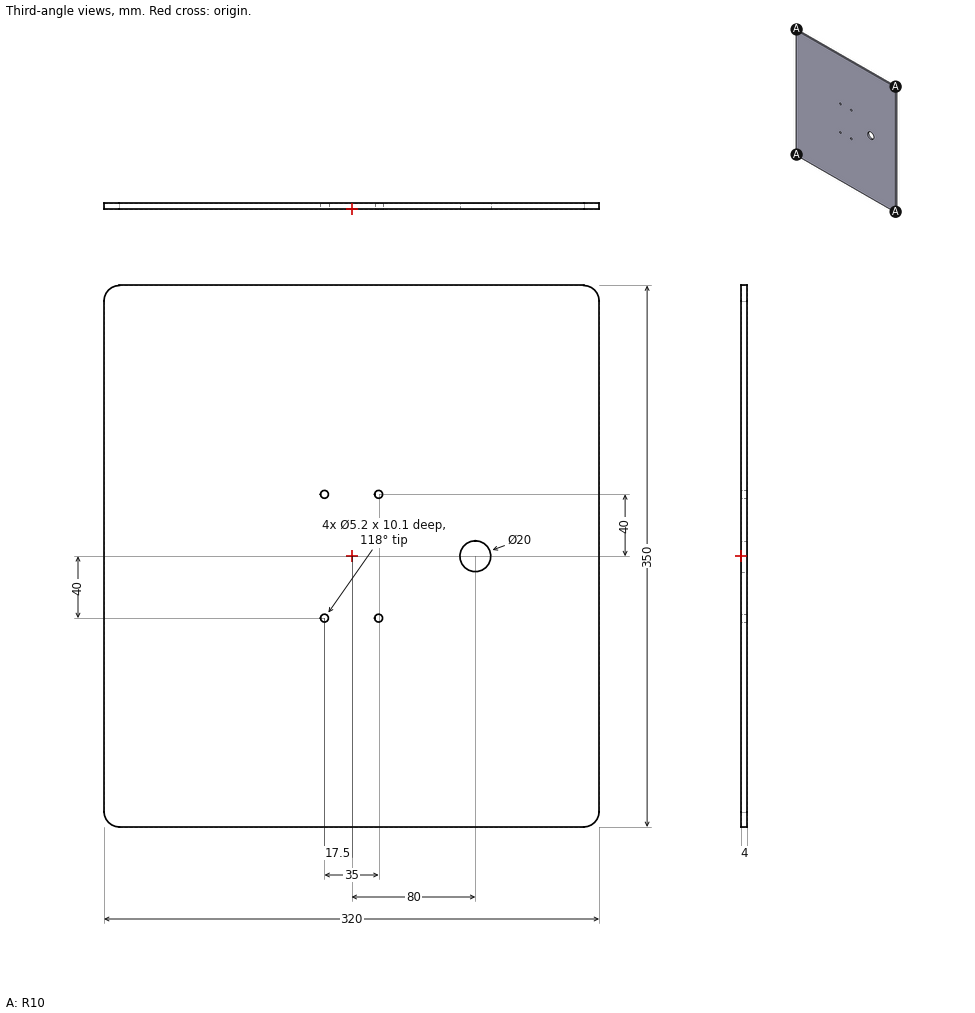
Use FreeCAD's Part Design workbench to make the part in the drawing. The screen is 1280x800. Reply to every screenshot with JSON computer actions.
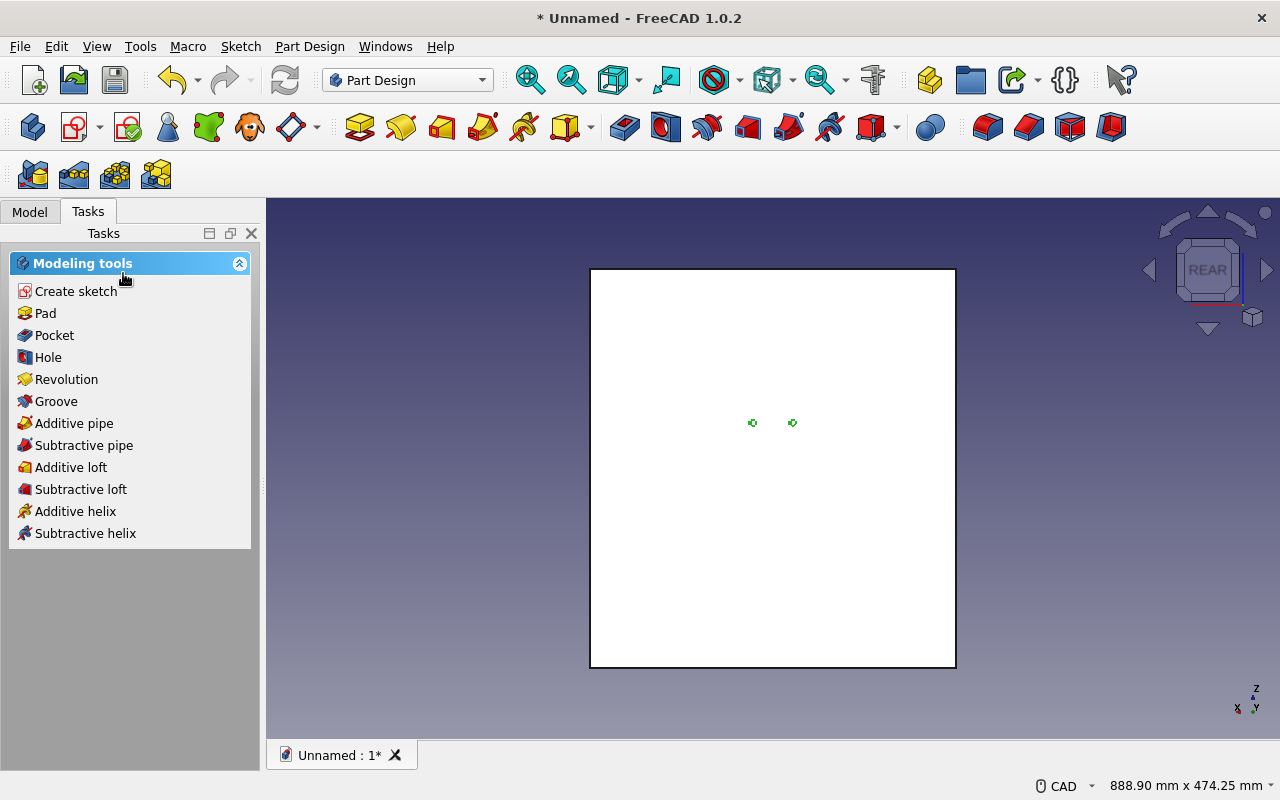
{"action": "left_click", "coordinate": [666, 128]}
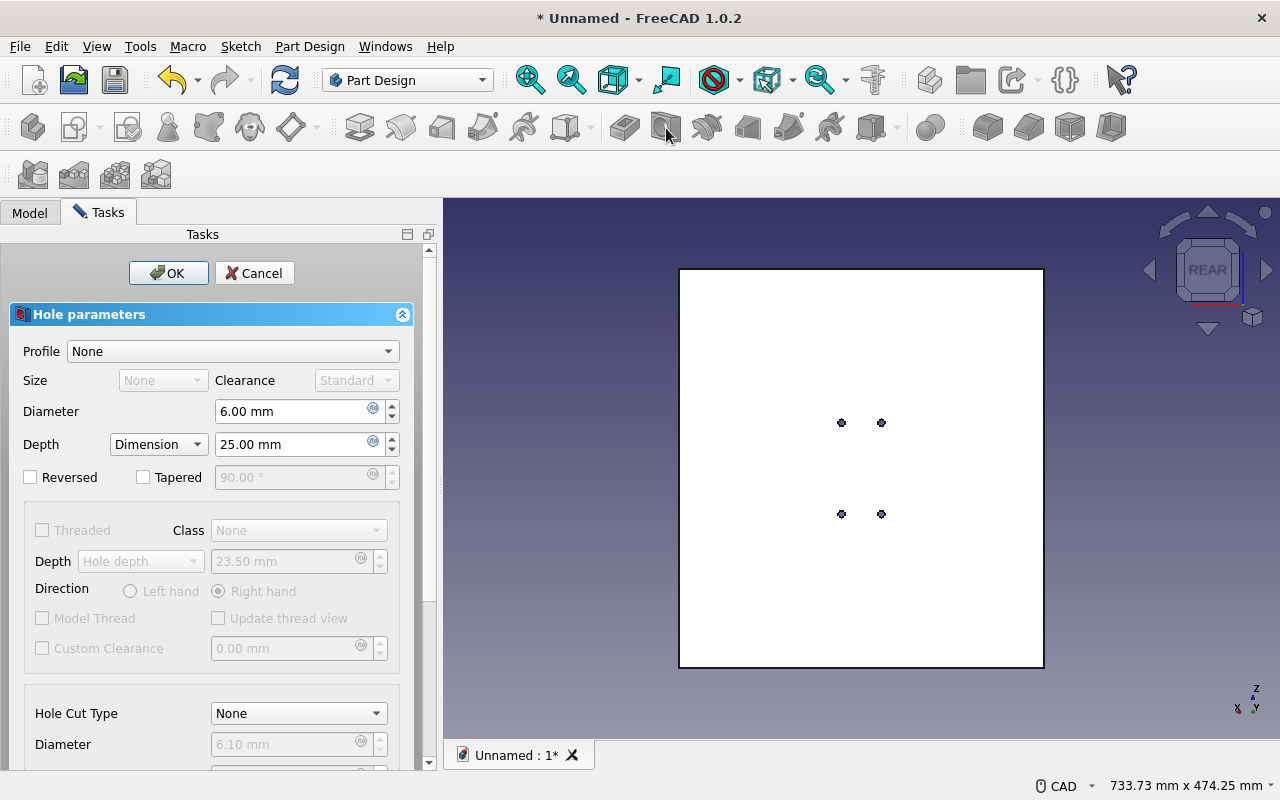
{"action": "triple_click", "coordinate": [300, 412]}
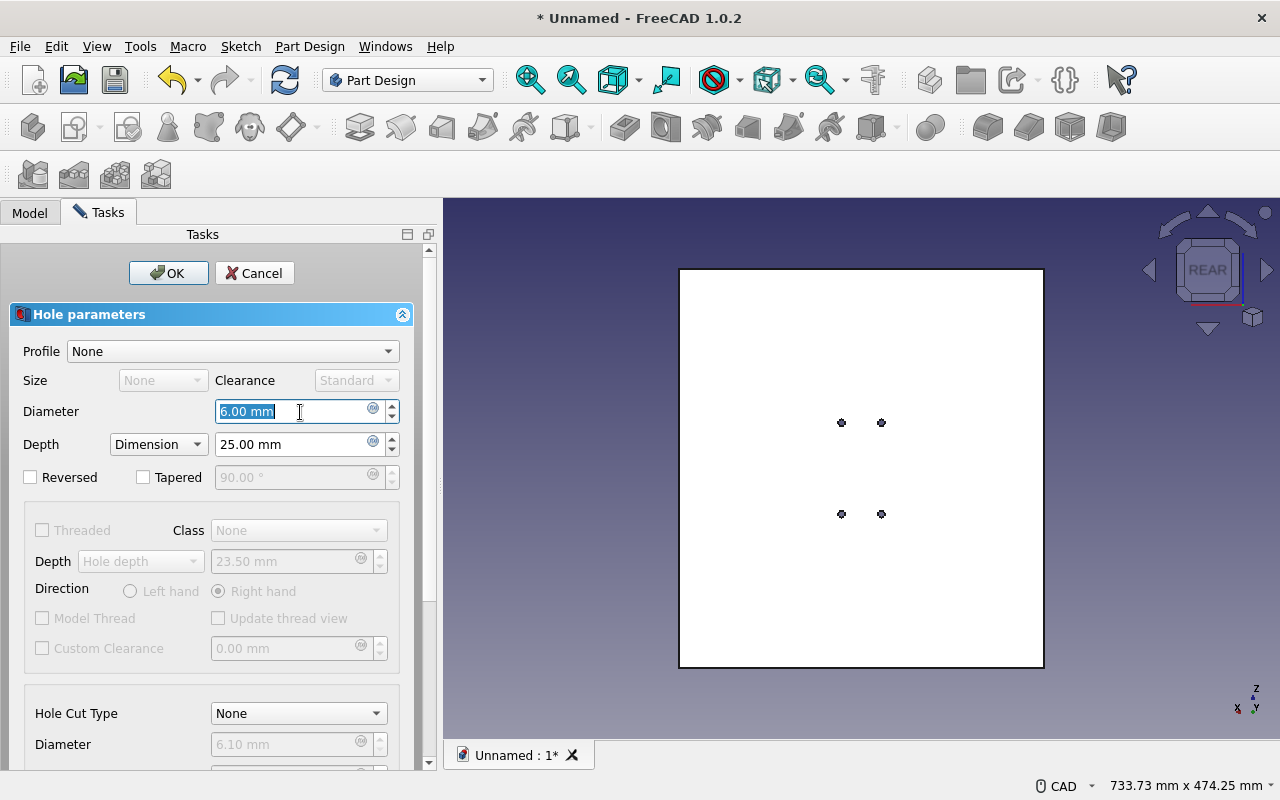
{"action": "type", "text": "5.2"}
{"action": "key", "text": "Tab"}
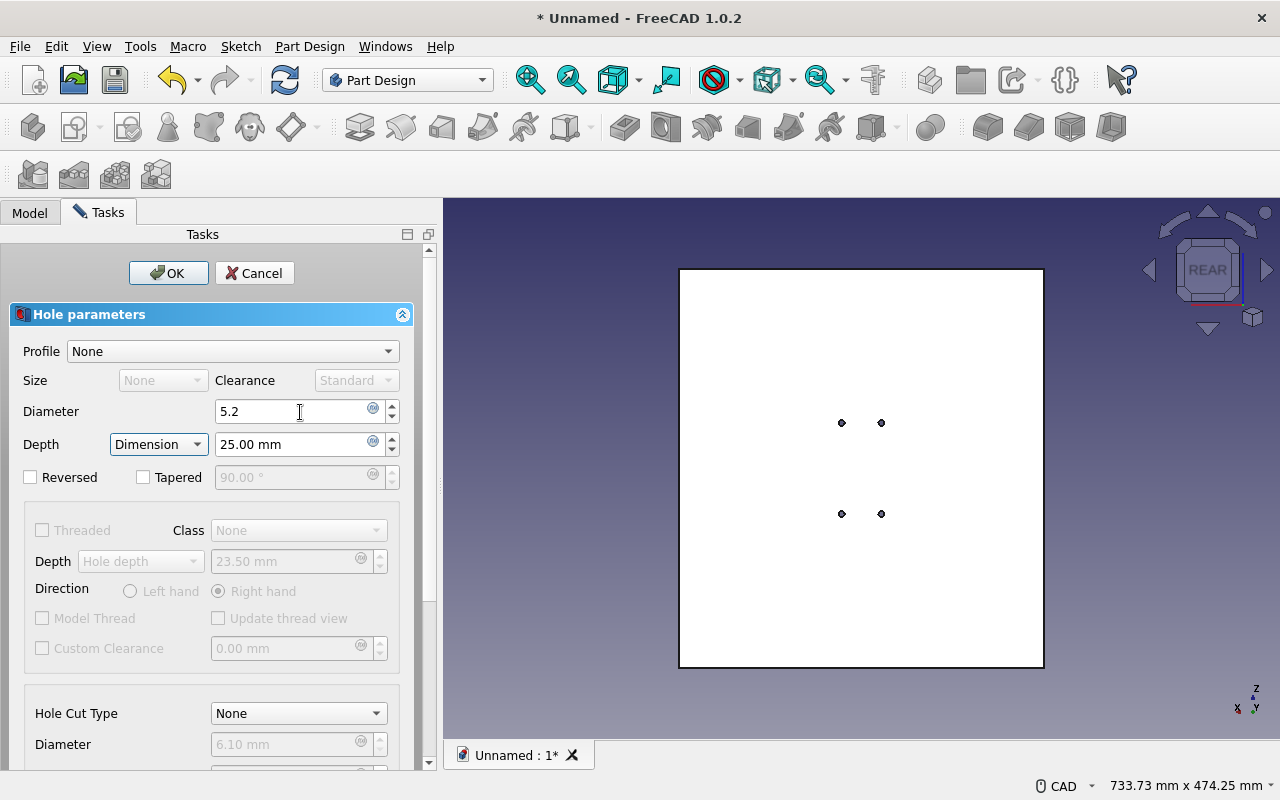
{"action": "triple_click", "coordinate": [300, 444]}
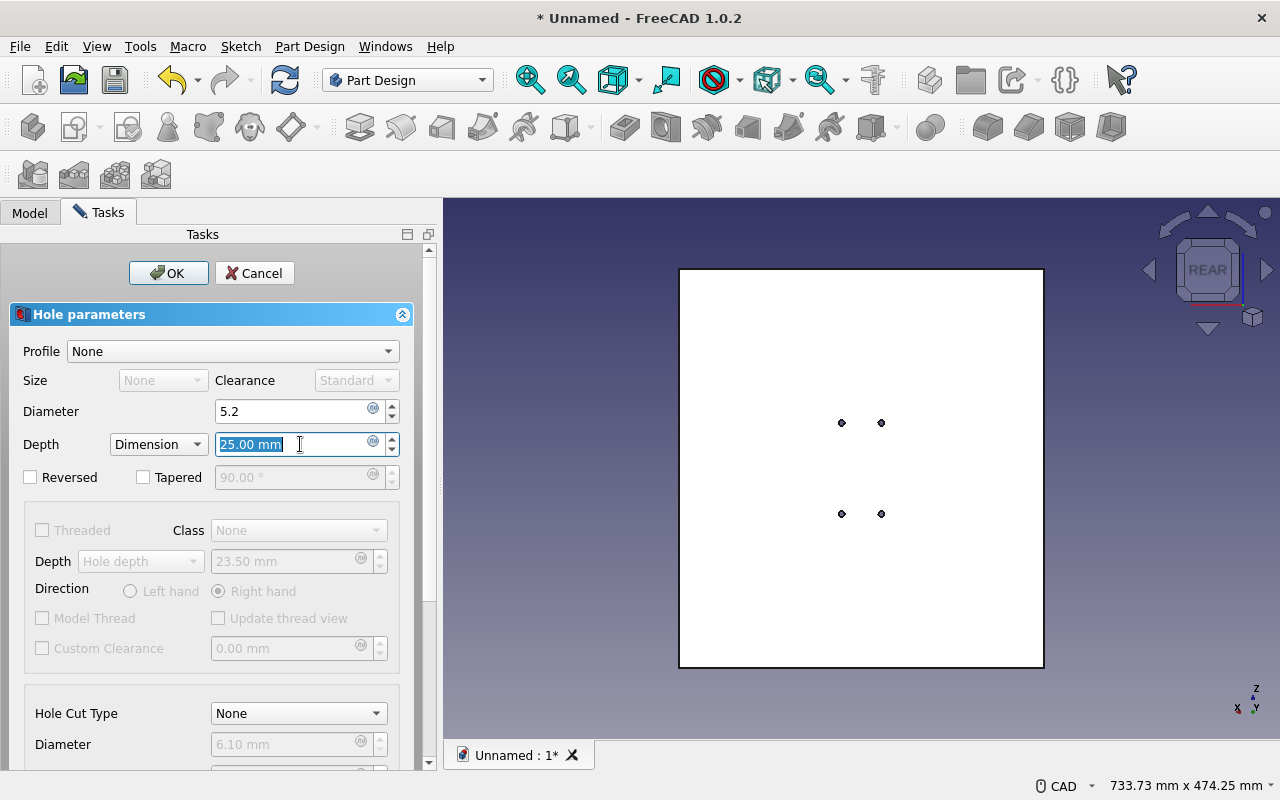
{"action": "type", "text": "10.1"}
{"action": "key", "text": "Tab"}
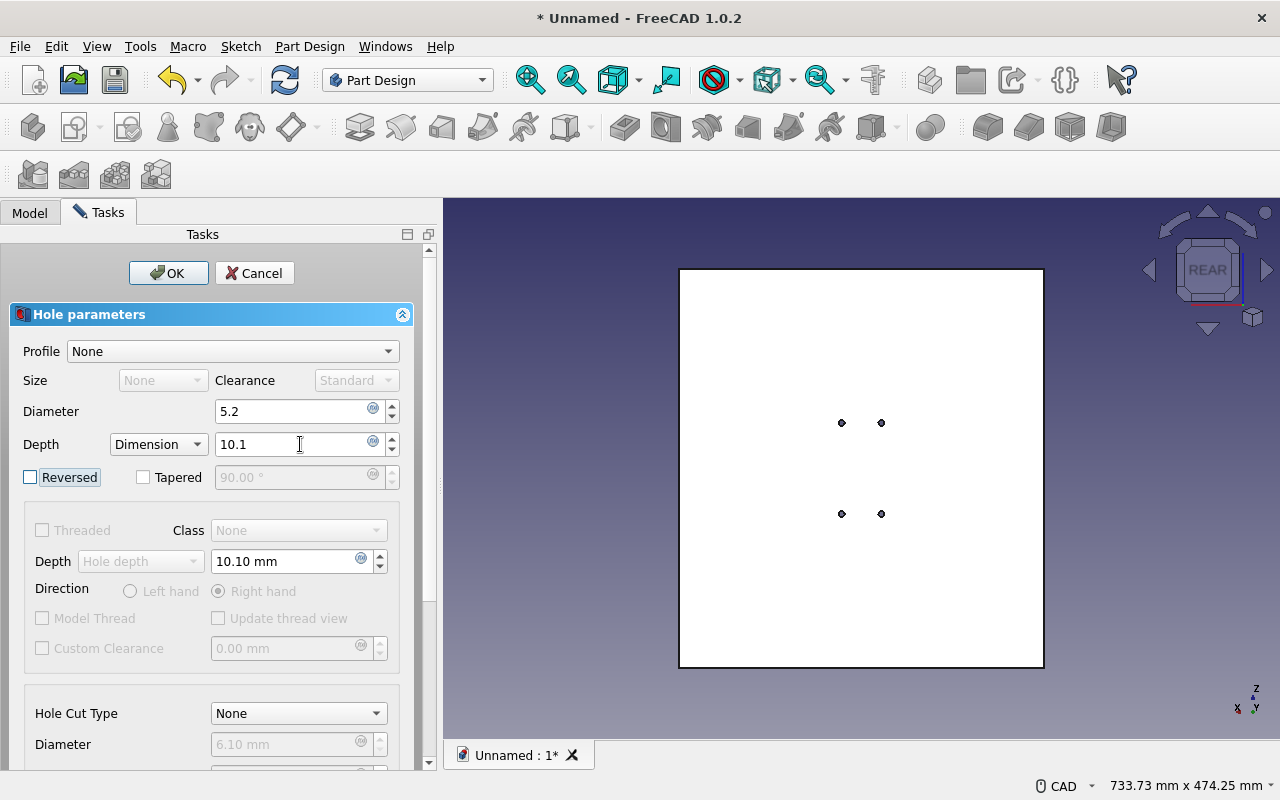
{"action": "left_click", "coordinate": [169, 273]}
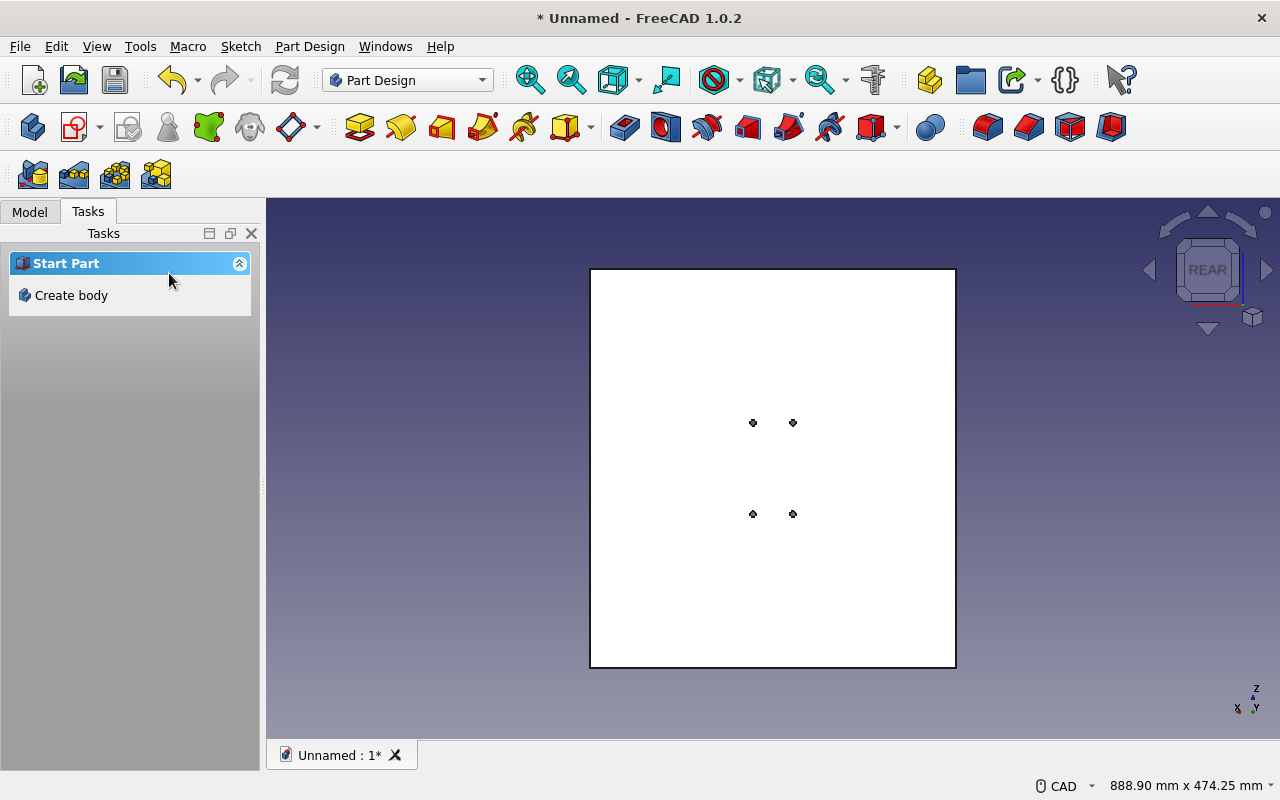
{"action": "scroll", "coordinate": [956, 667], "scroll_direction": "up", "scroll_amount": 11}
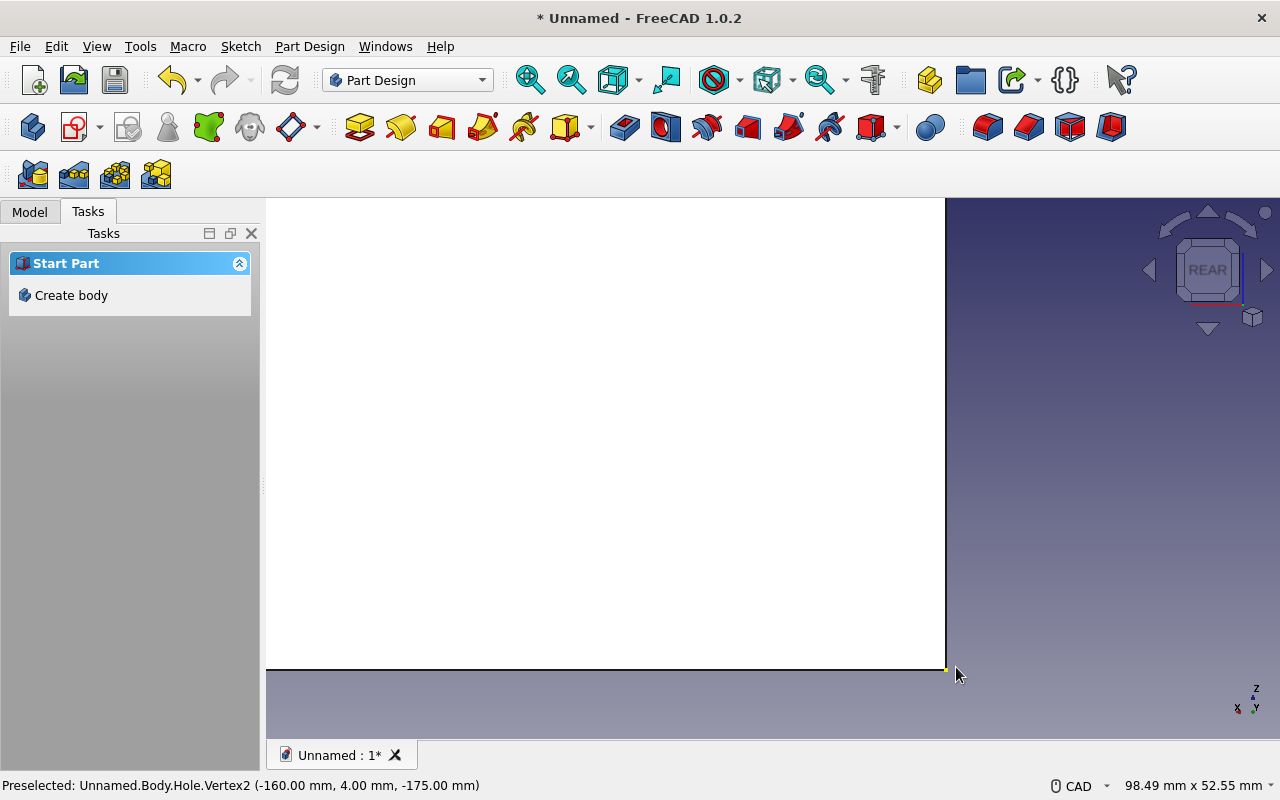
{"action": "left_click", "coordinate": [531, 80]}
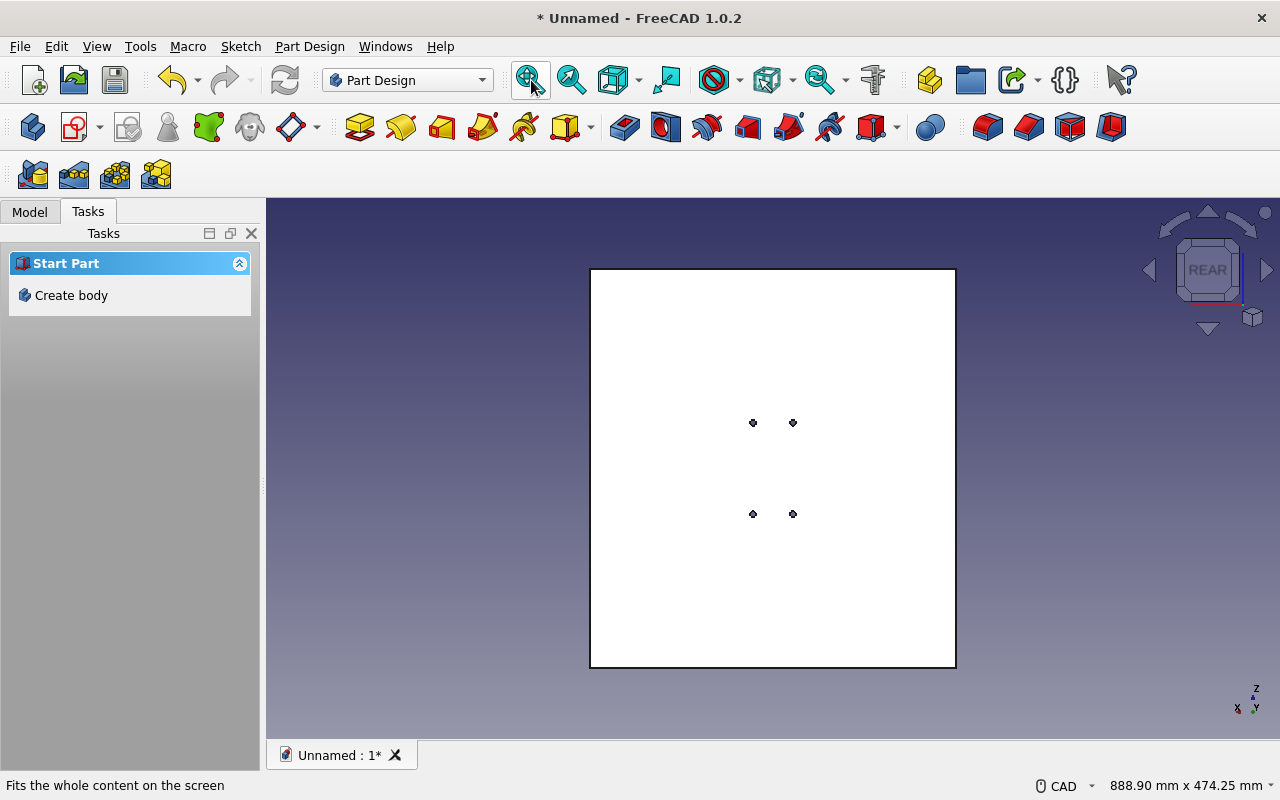
{"action": "key", "text": "0"}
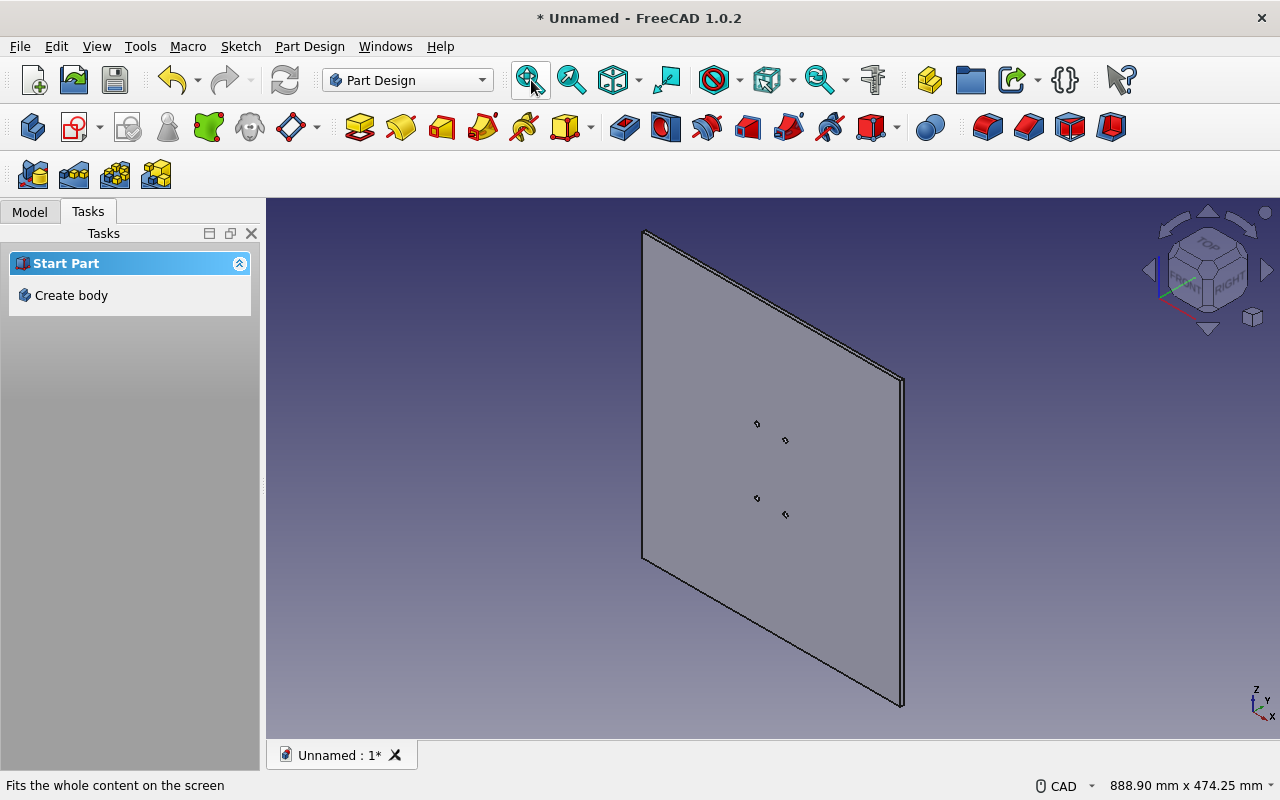
{"action": "scroll", "coordinate": [644, 556], "scroll_direction": "up", "scroll_amount": 11}